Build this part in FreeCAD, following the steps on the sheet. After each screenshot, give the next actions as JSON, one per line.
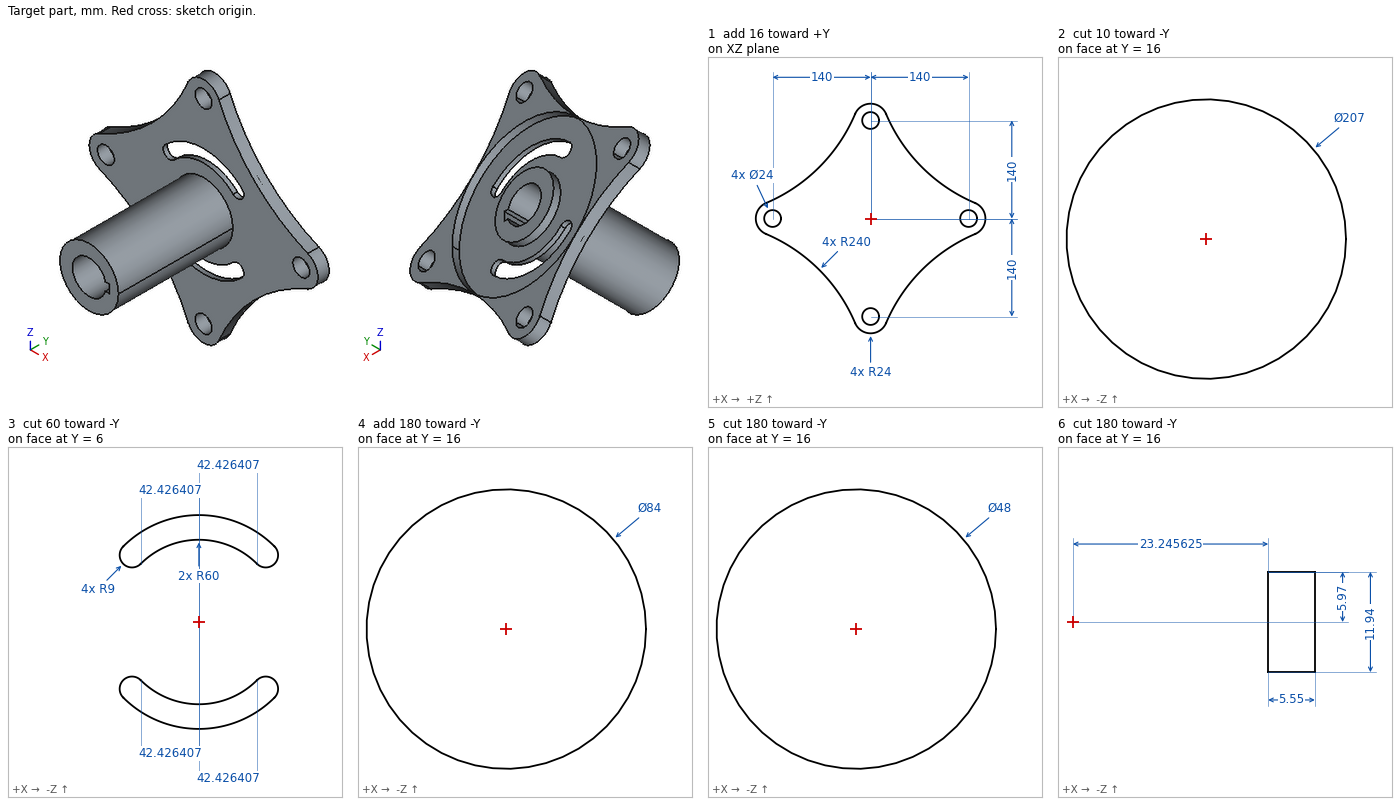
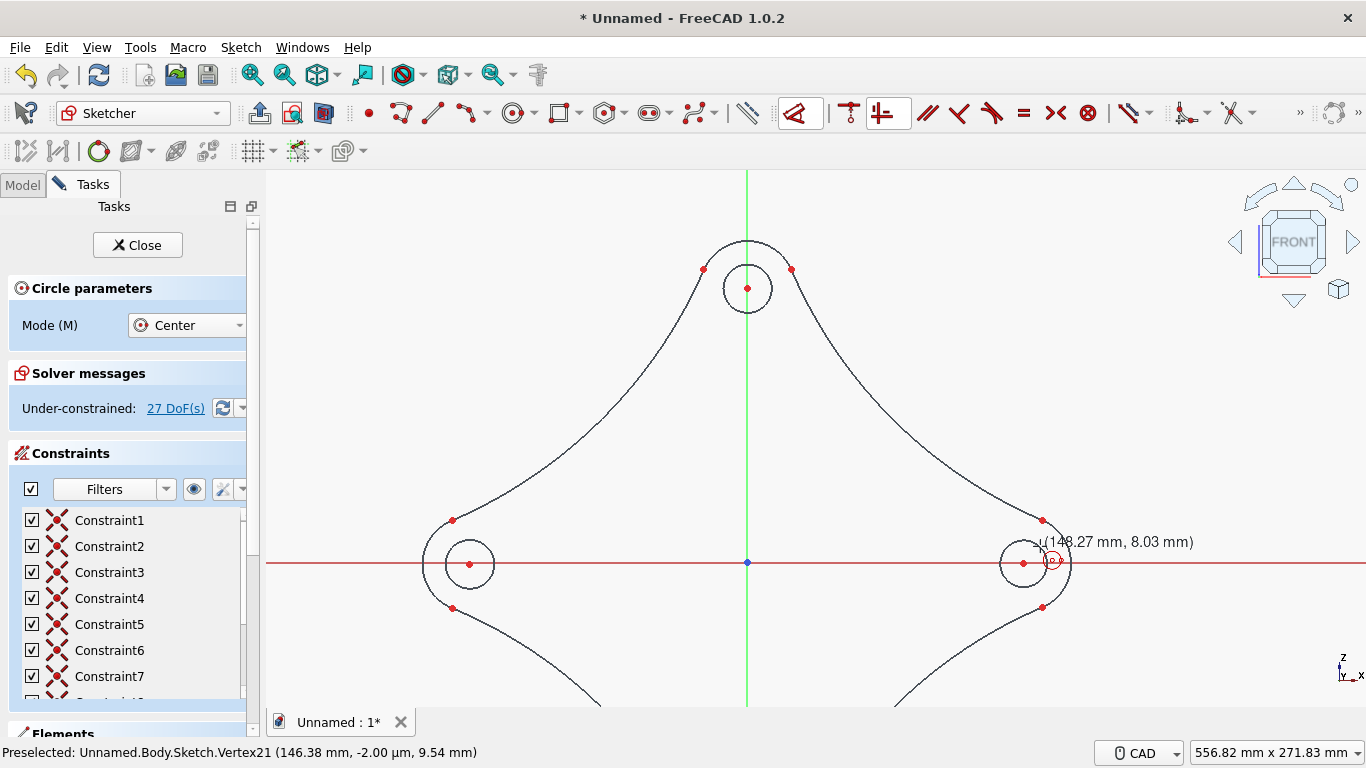
{"action": "scroll", "coordinate": [748, 287], "scroll_direction": "down", "scroll_amount": 3}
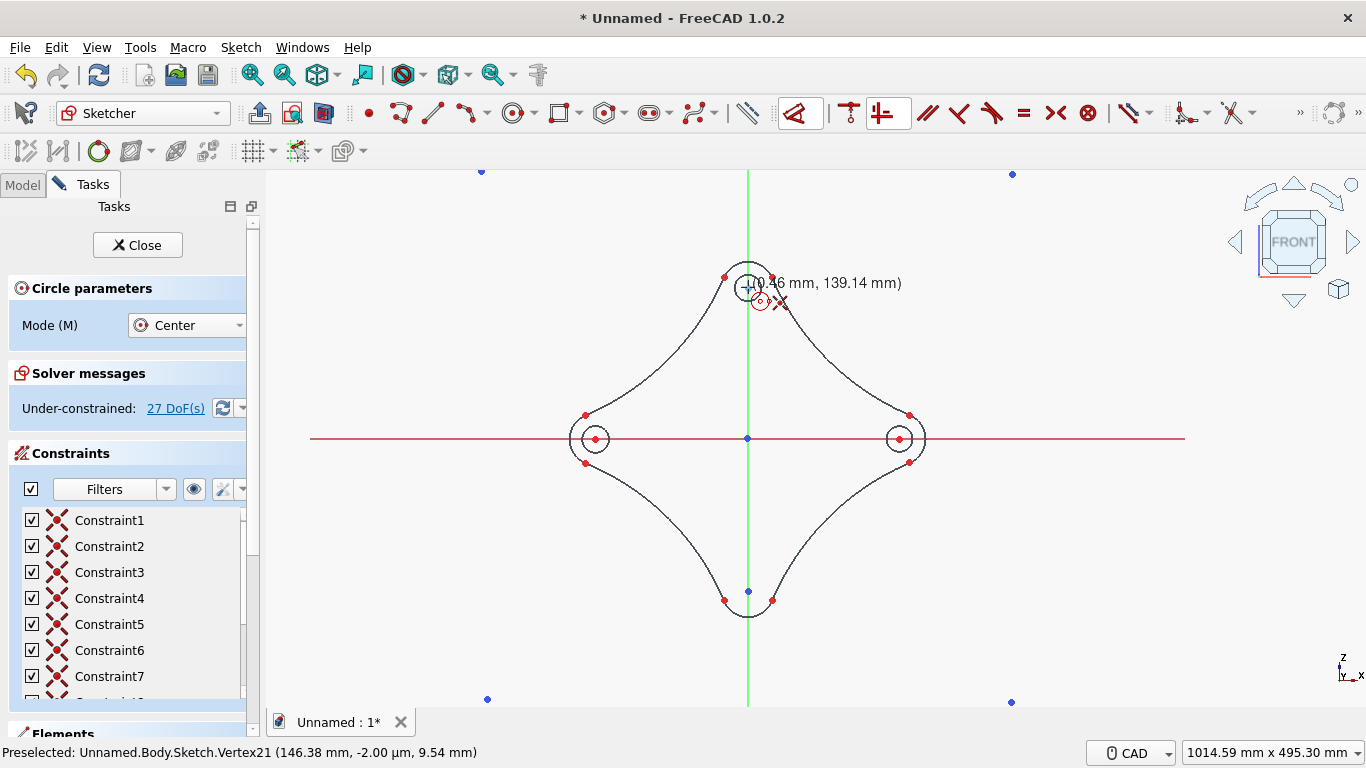
{"action": "scroll", "coordinate": [748, 590], "scroll_direction": "up", "scroll_amount": 3}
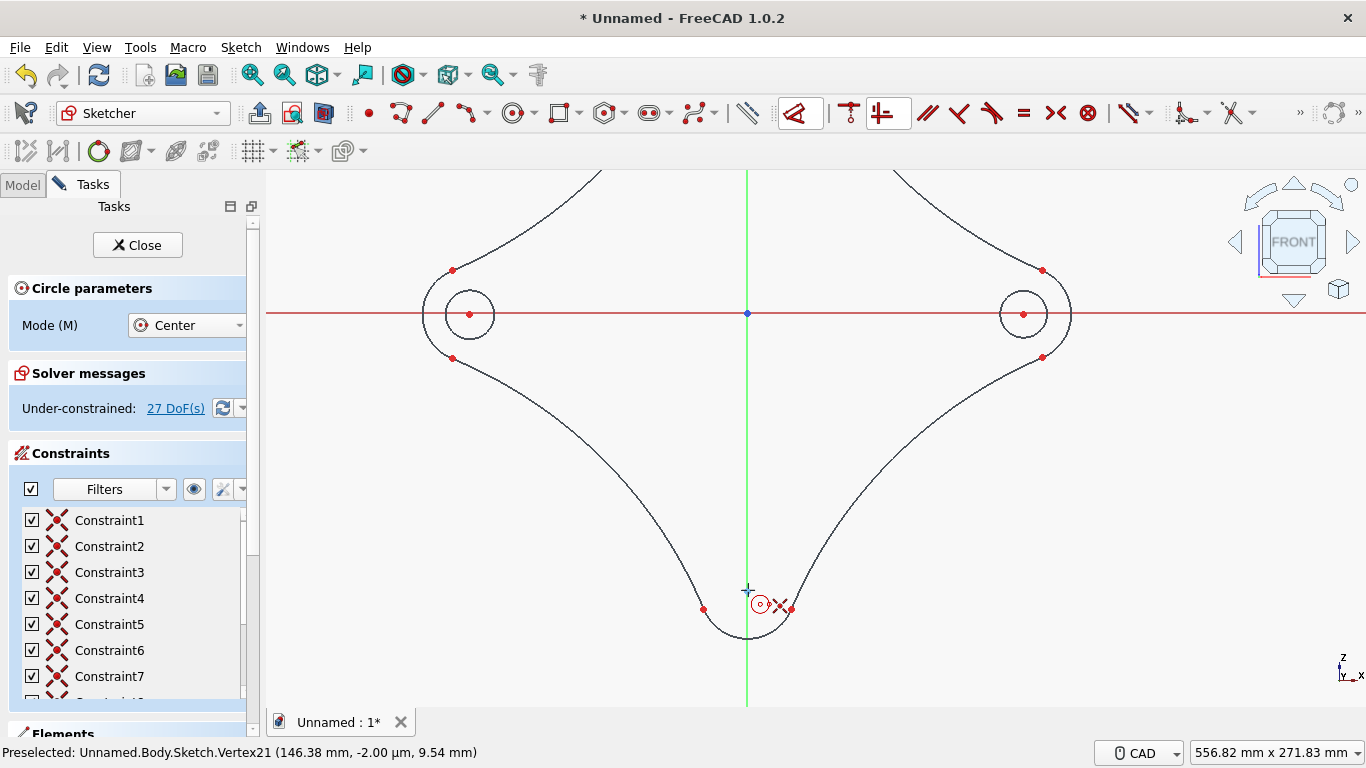
{"action": "left_click", "coordinate": [747, 590]}
{"action": "left_click", "coordinate": [764, 573]}
{"action": "key", "text": "Escape"}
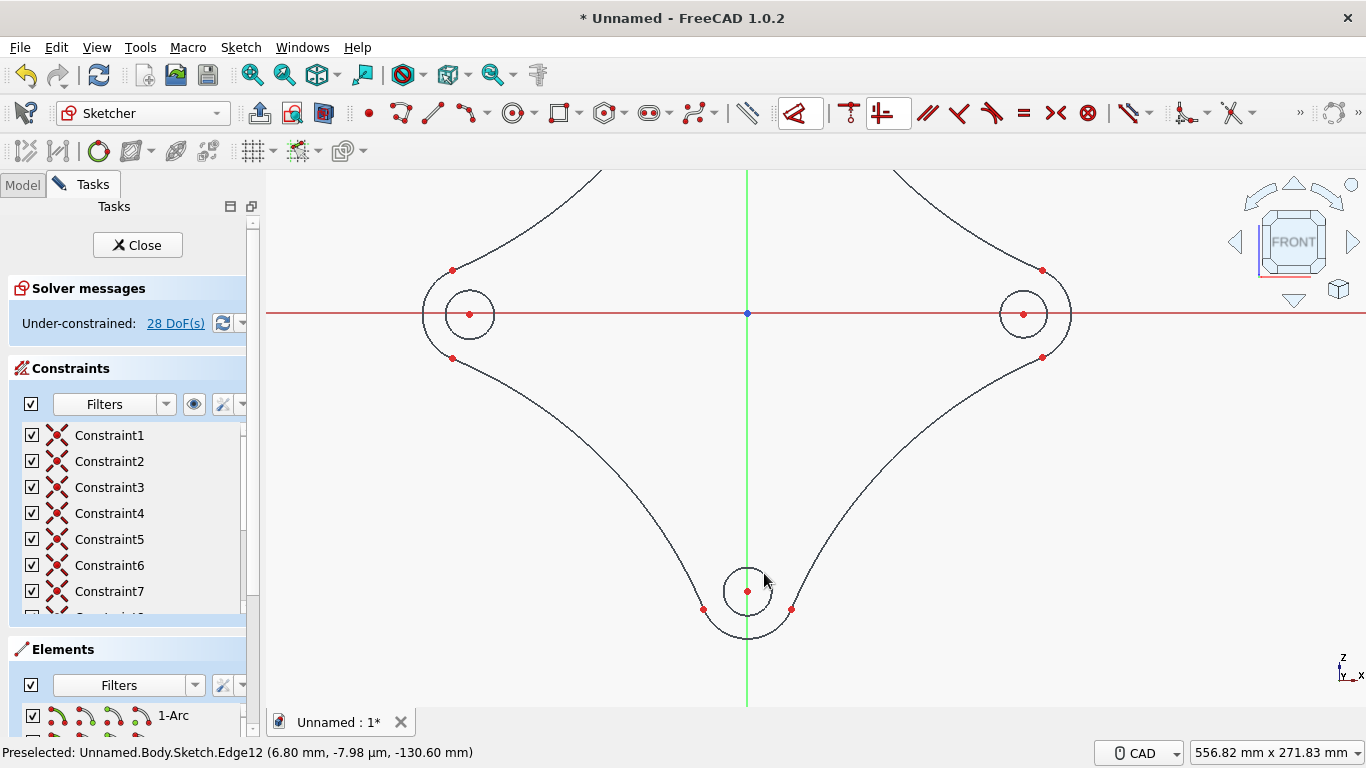
{"action": "left_click", "coordinate": [726, 634]}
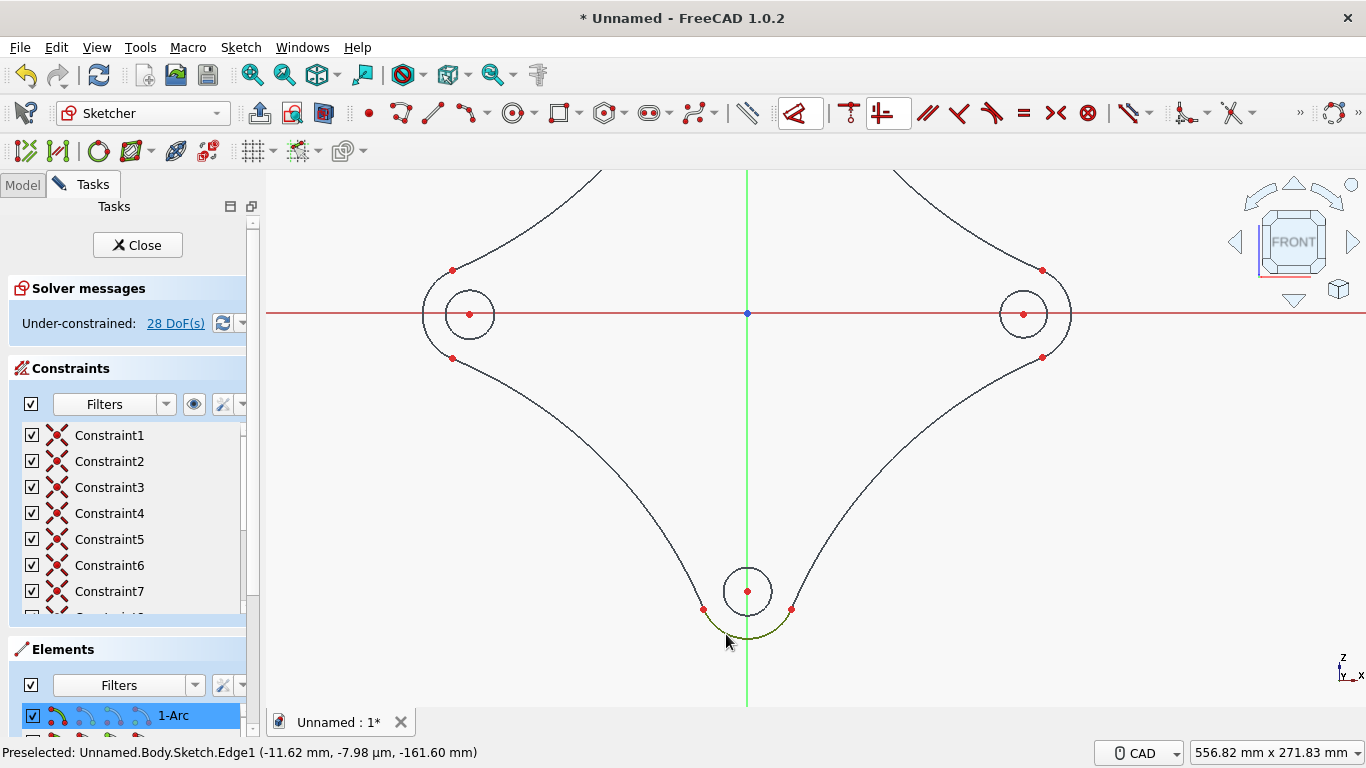
{"action": "left_click", "coordinate": [650, 514]}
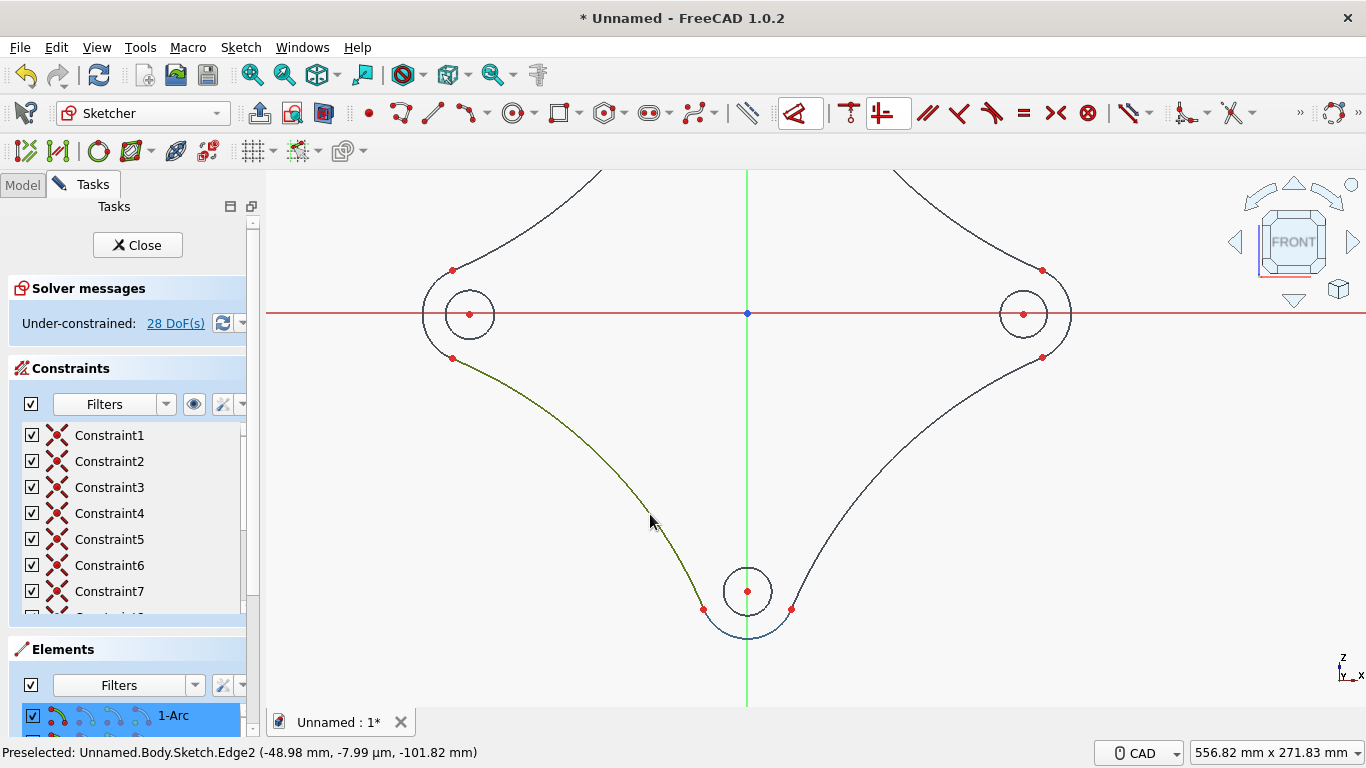
{"action": "left_click", "coordinate": [992, 114]}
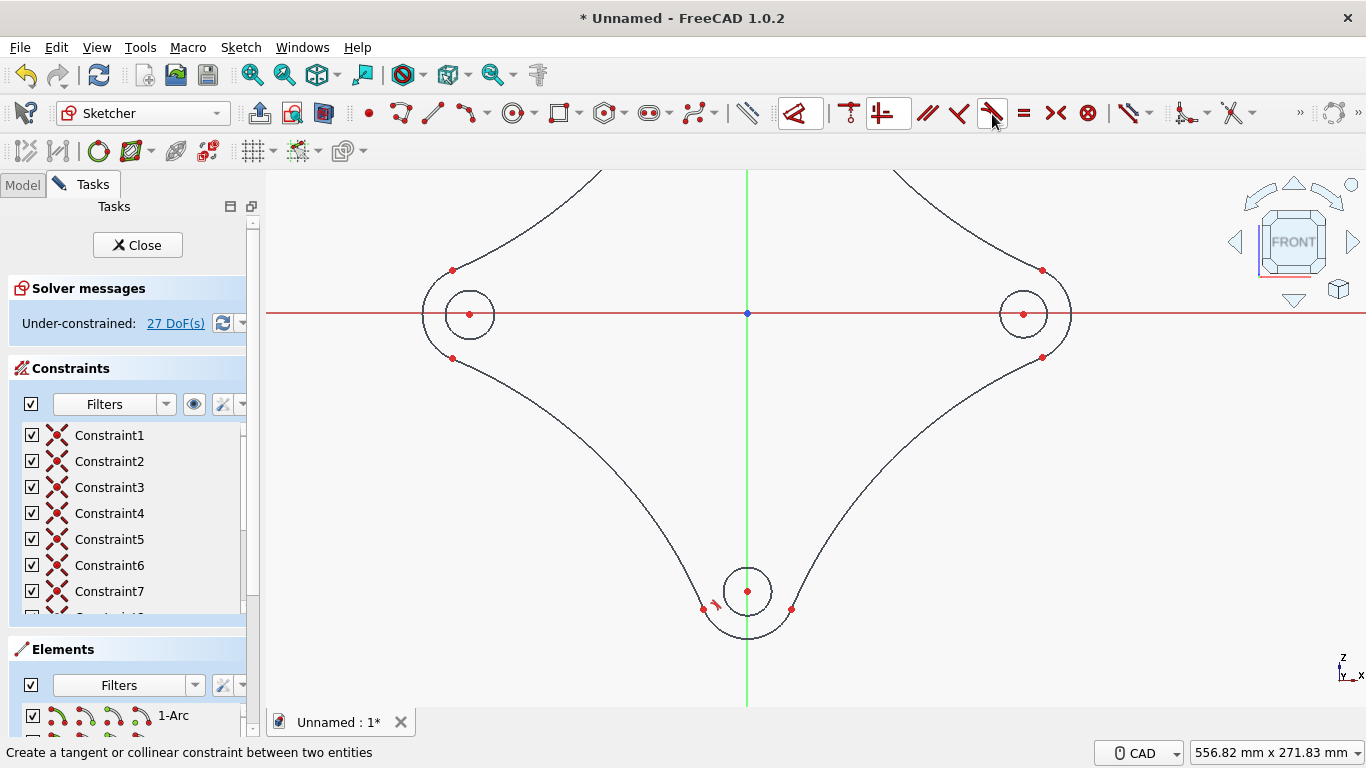
{"action": "left_click", "coordinate": [726, 634]}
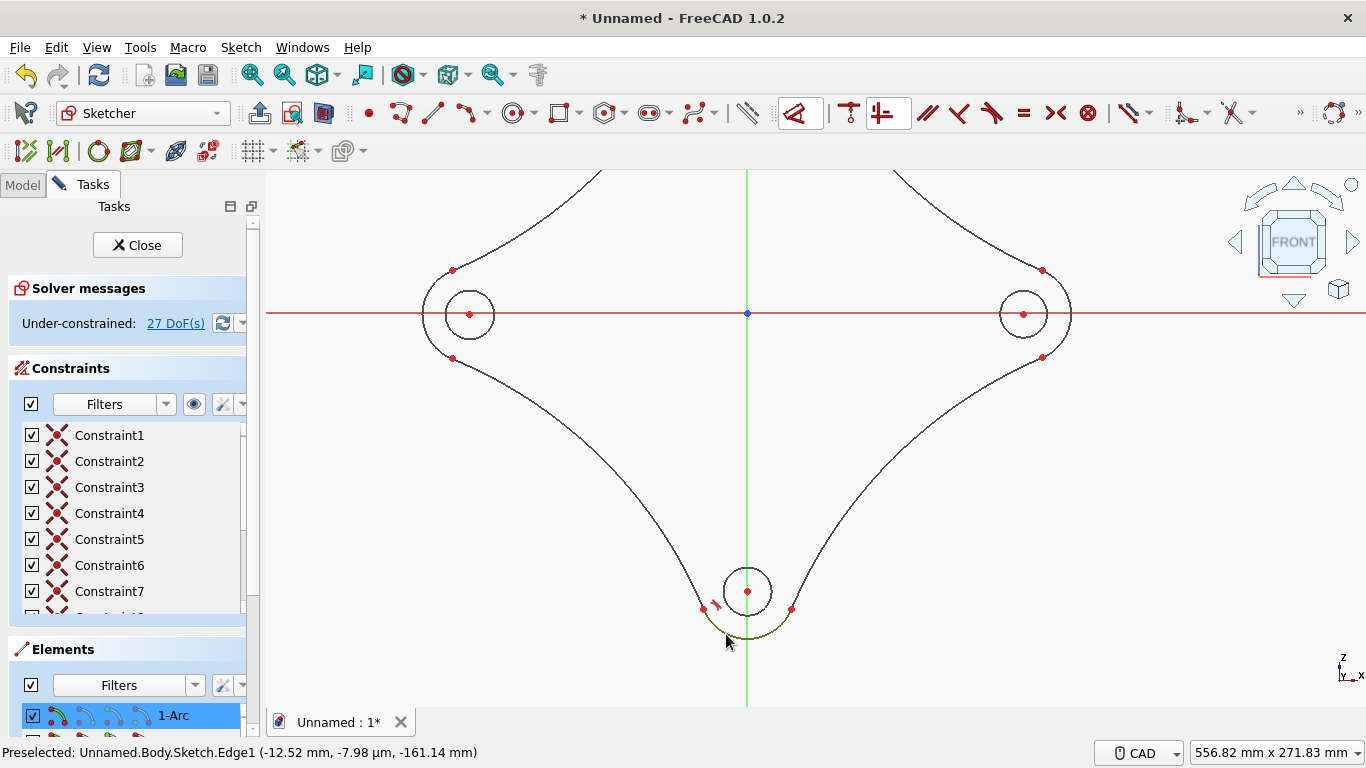
{"action": "left_click", "coordinate": [948, 412]}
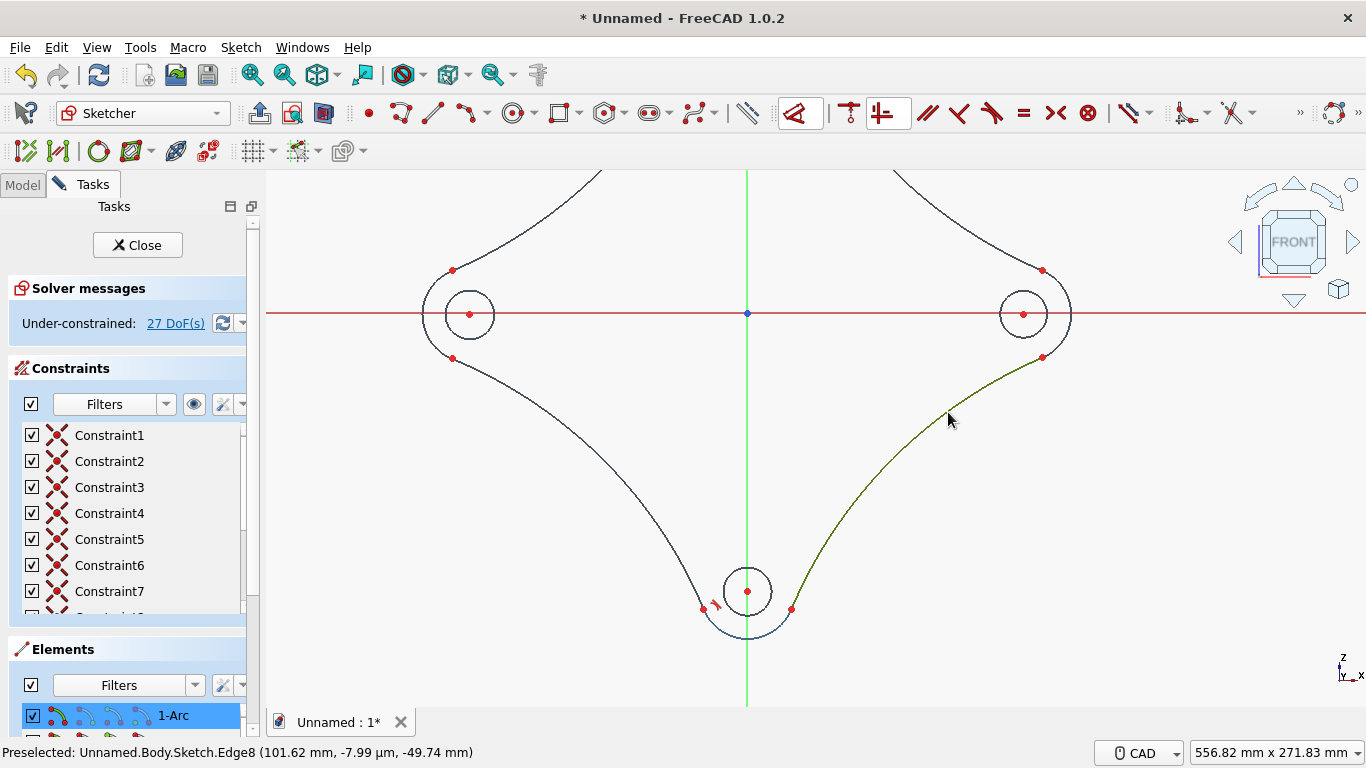
{"action": "left_click", "coordinate": [992, 114]}